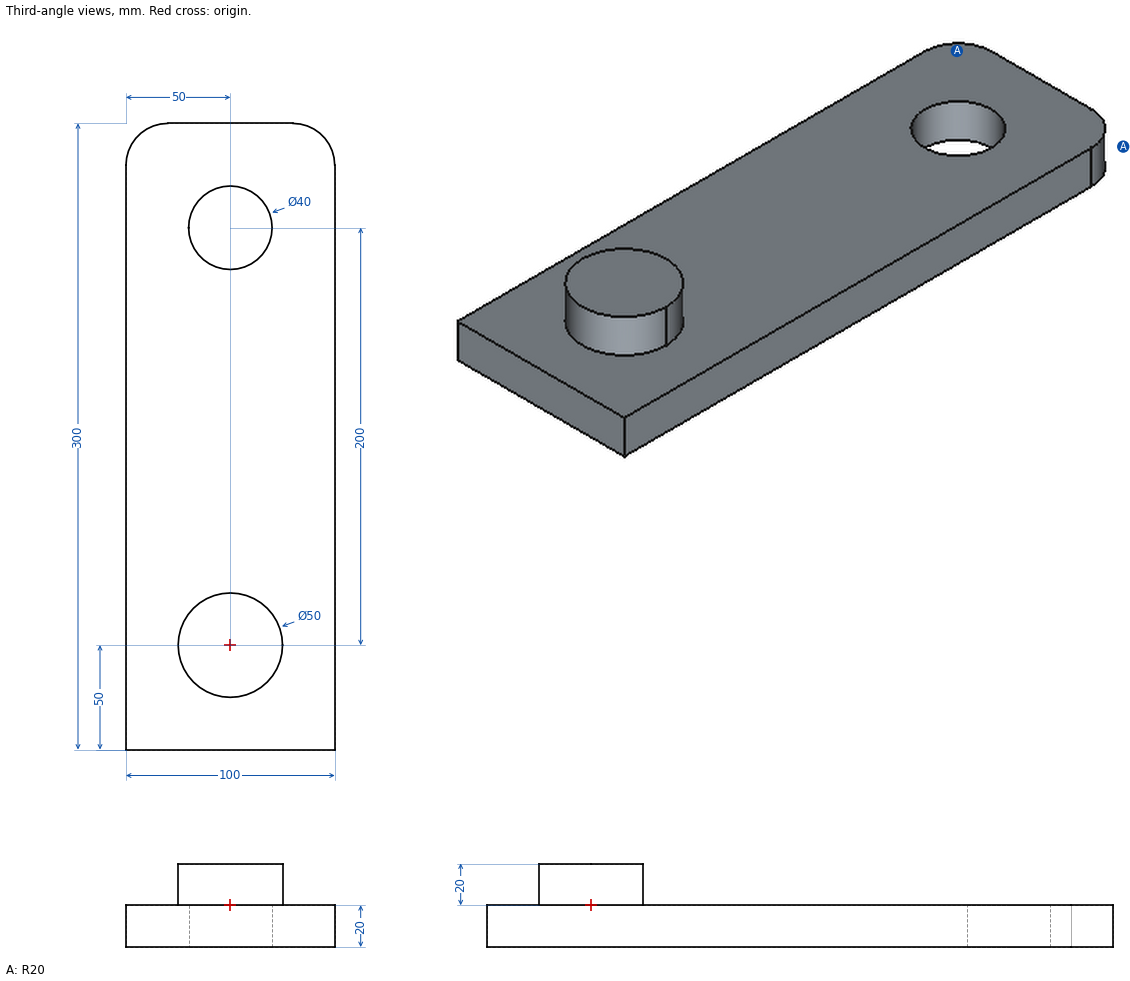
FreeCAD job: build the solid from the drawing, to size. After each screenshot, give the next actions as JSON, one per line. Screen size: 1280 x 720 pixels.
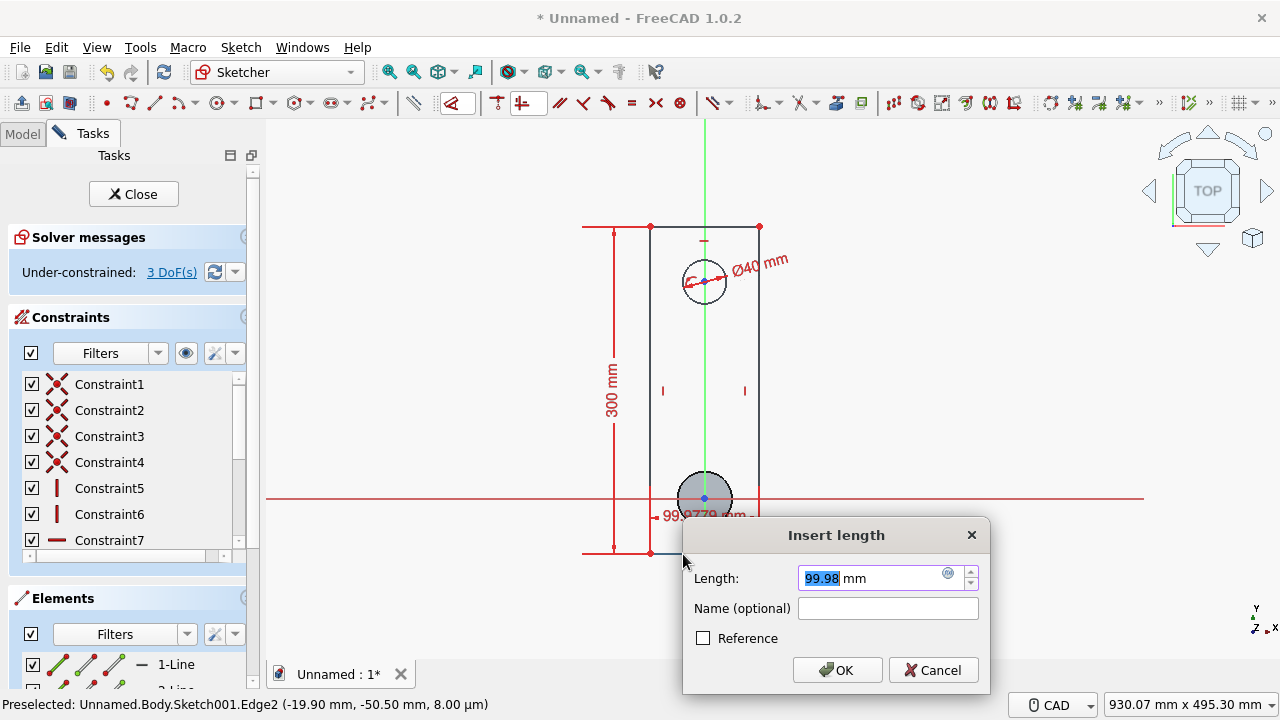
{"action": "type", "text": "100"}
{"action": "key", "text": "Return"}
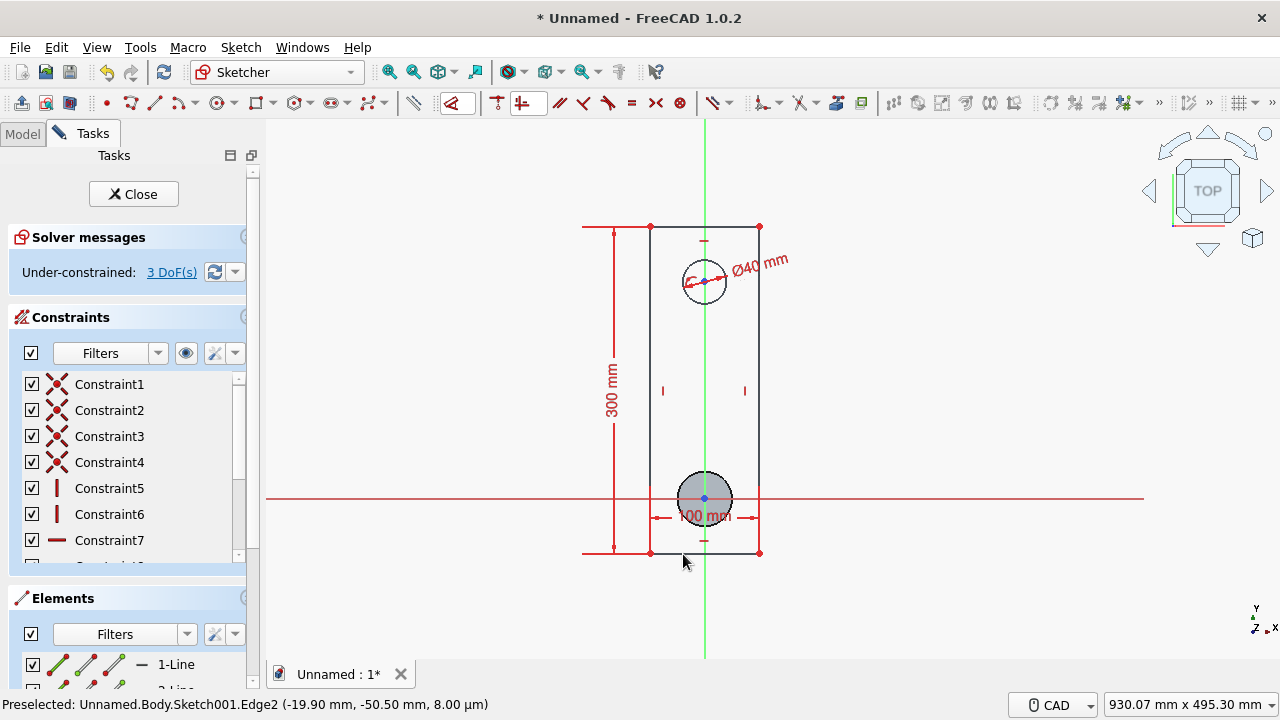
{"action": "left_click", "coordinate": [650, 227]}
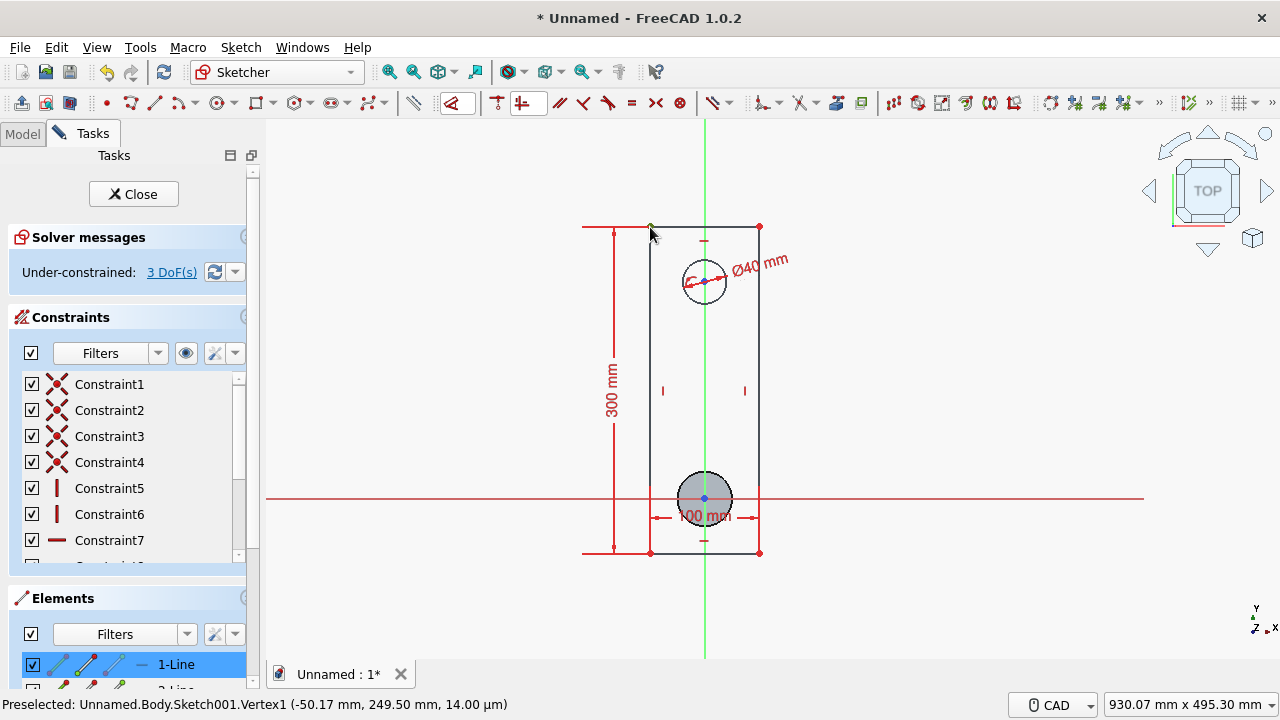
{"action": "left_click", "coordinate": [470, 104]}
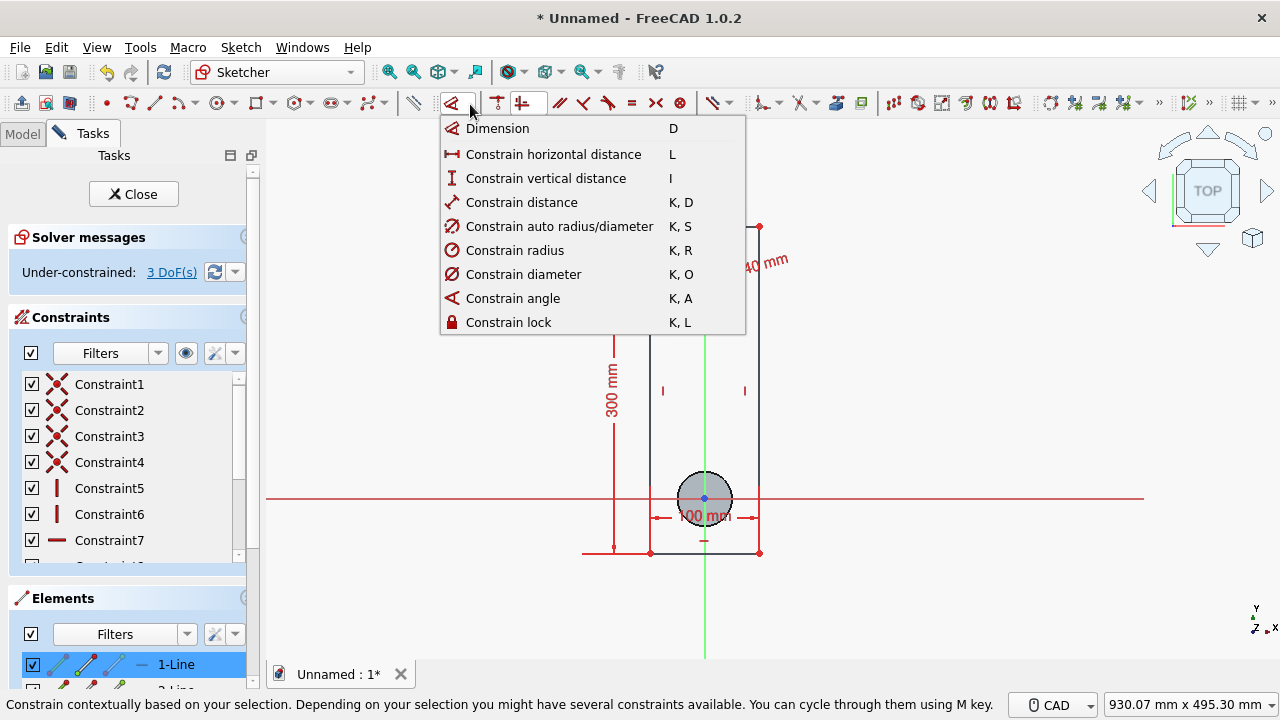
{"action": "left_click", "coordinate": [593, 154]}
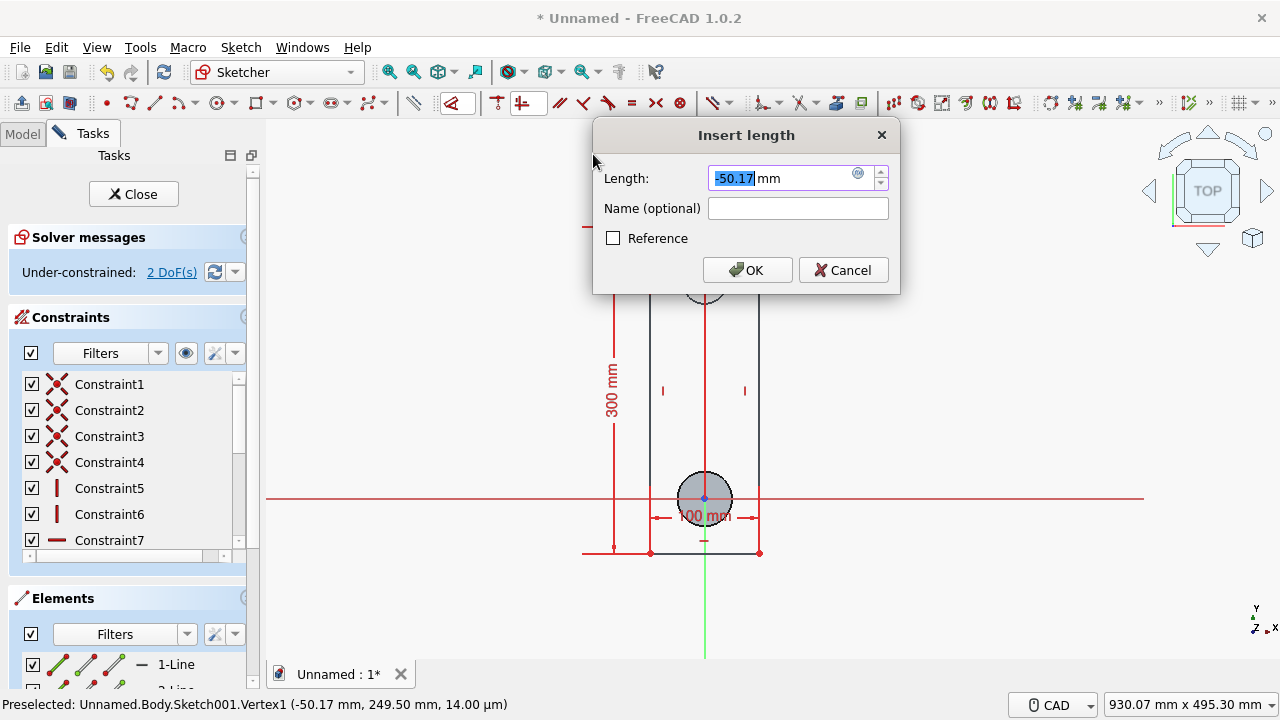
{"action": "type", "text": "-50"}
{"action": "key", "text": "Return"}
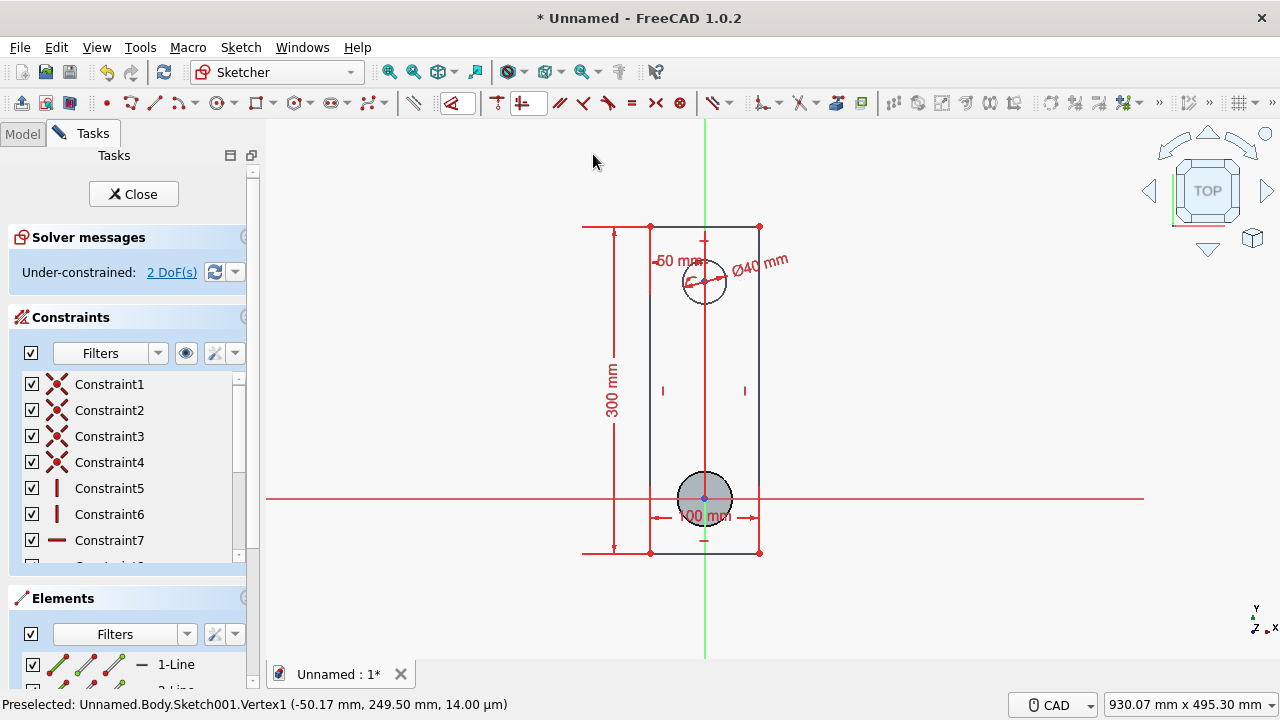
{"action": "left_click", "coordinate": [650, 554]}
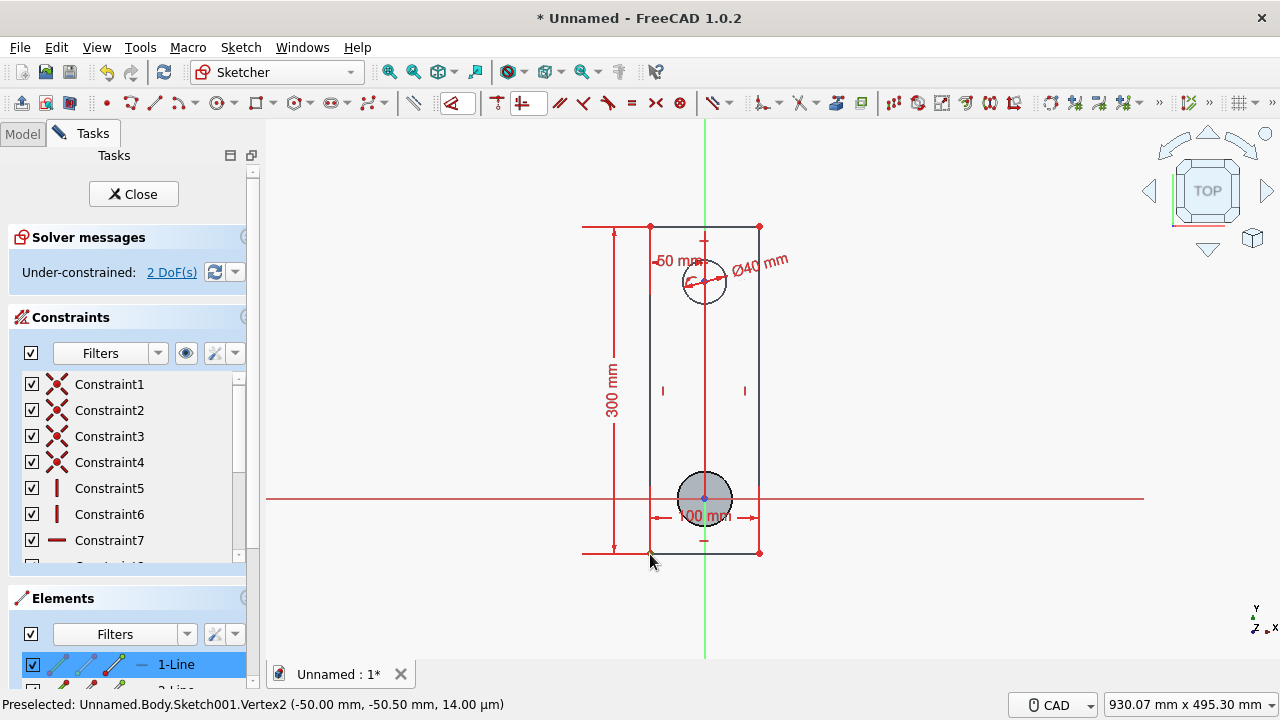
{"action": "left_click", "coordinate": [470, 104]}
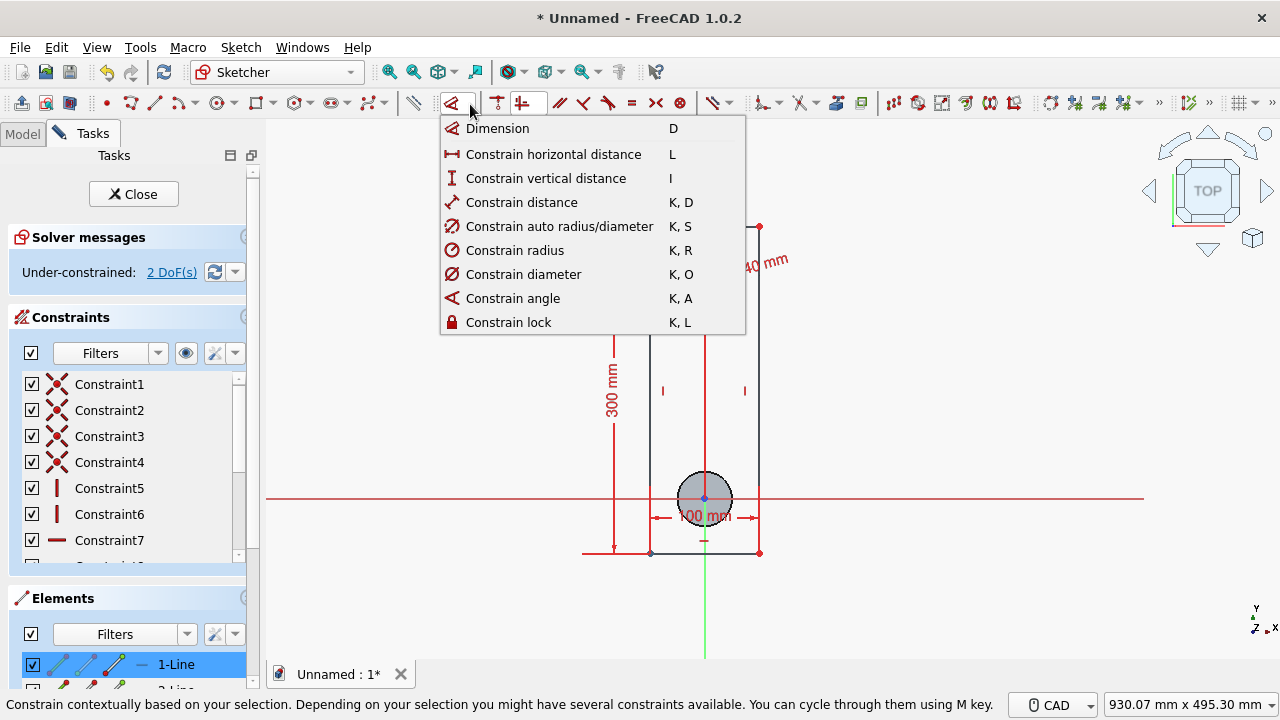
{"action": "left_click", "coordinate": [593, 178]}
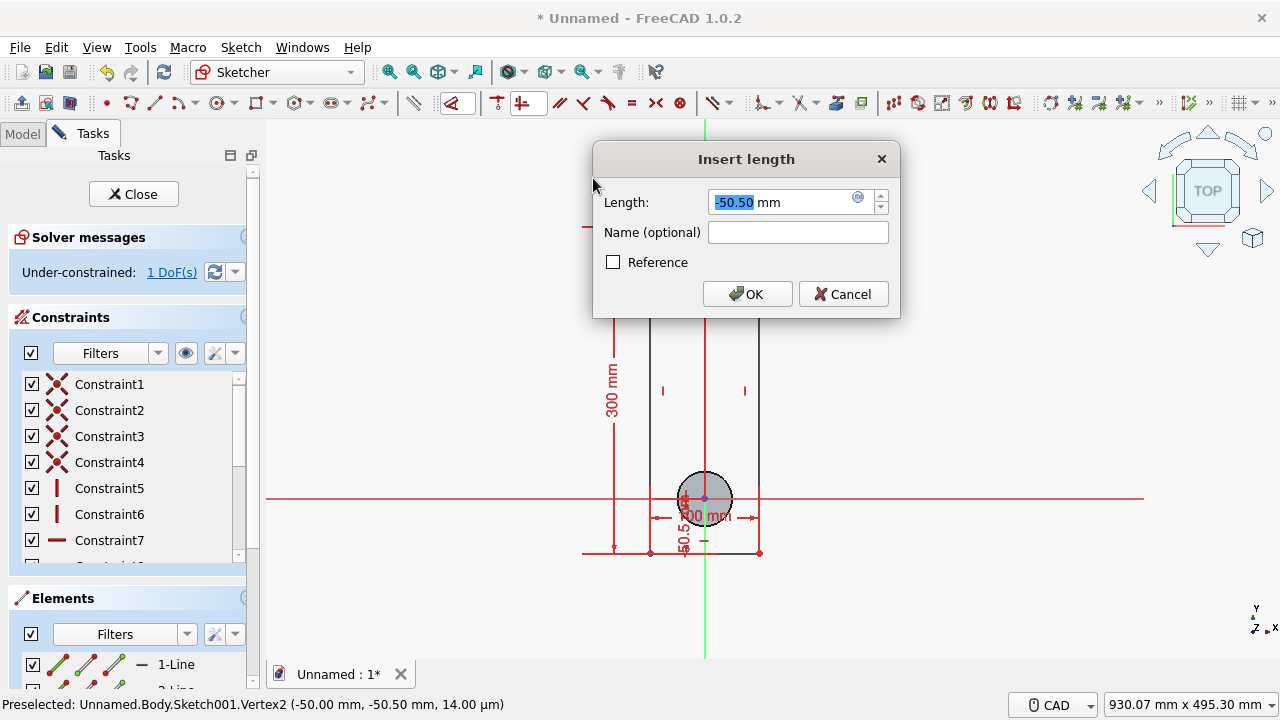
{"action": "type", "text": "-50"}
{"action": "key", "text": "Return"}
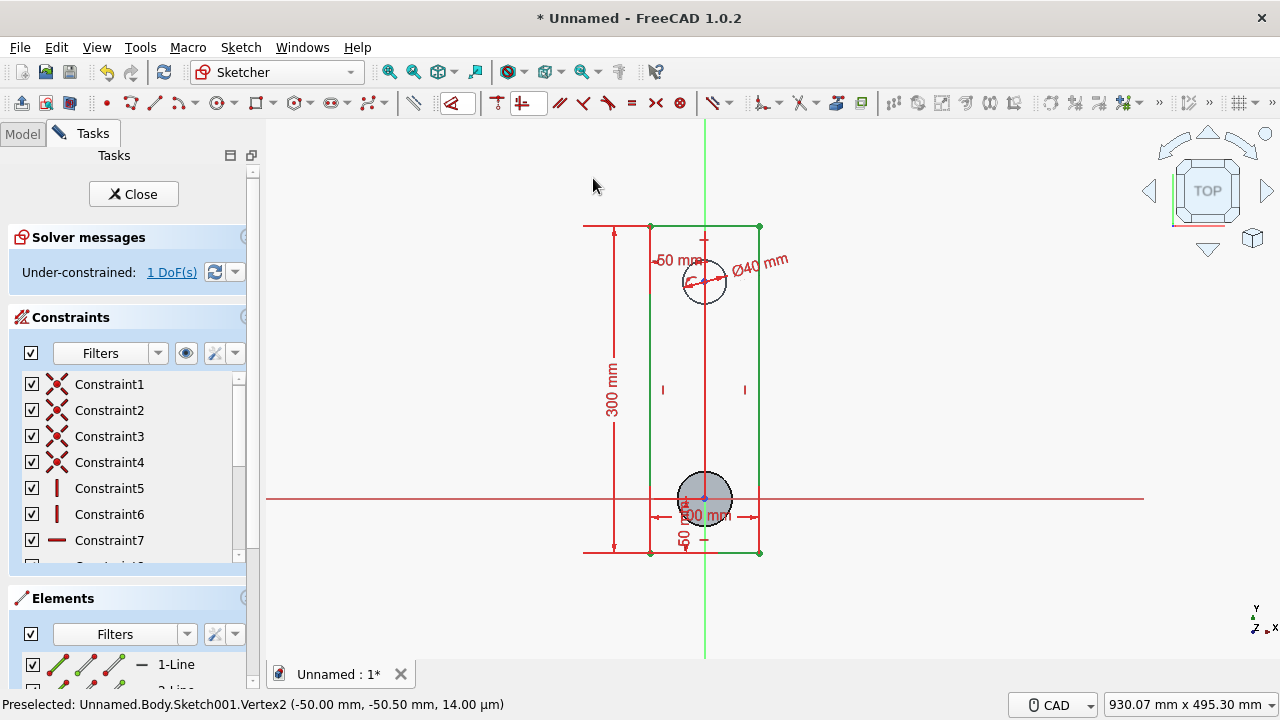
{"action": "left_click", "coordinate": [705, 282]}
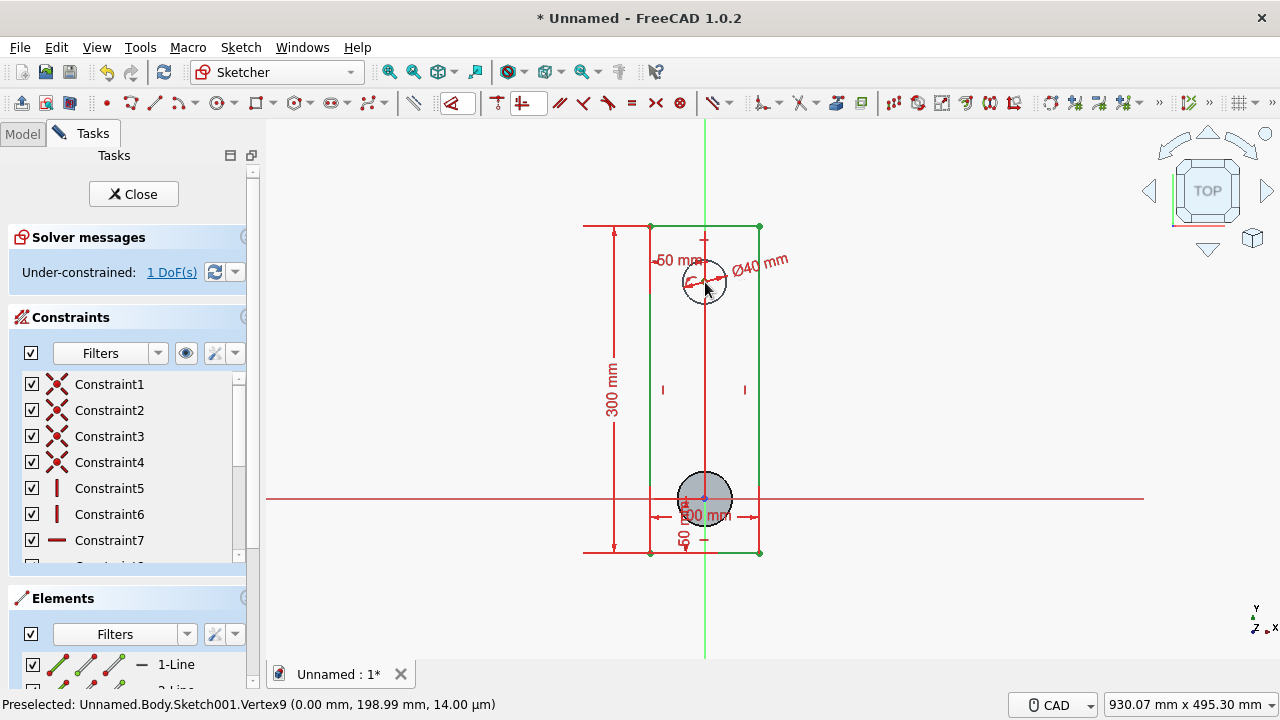
{"action": "left_click", "coordinate": [470, 104]}